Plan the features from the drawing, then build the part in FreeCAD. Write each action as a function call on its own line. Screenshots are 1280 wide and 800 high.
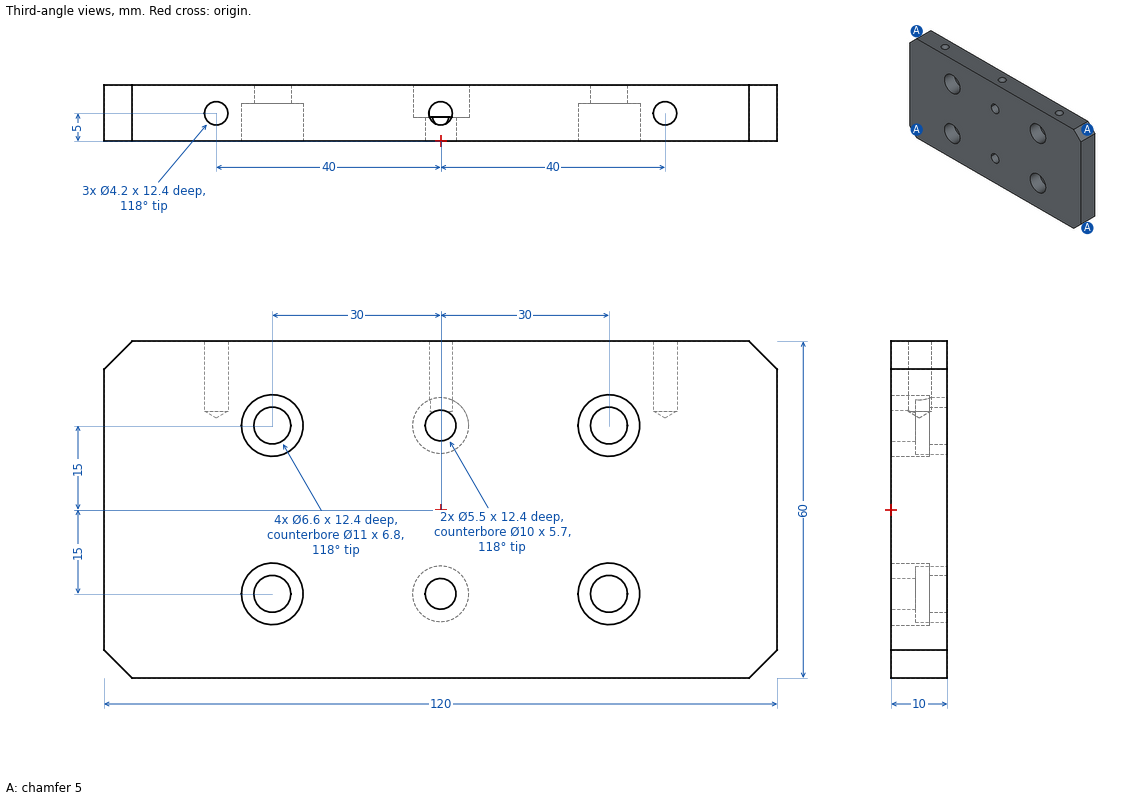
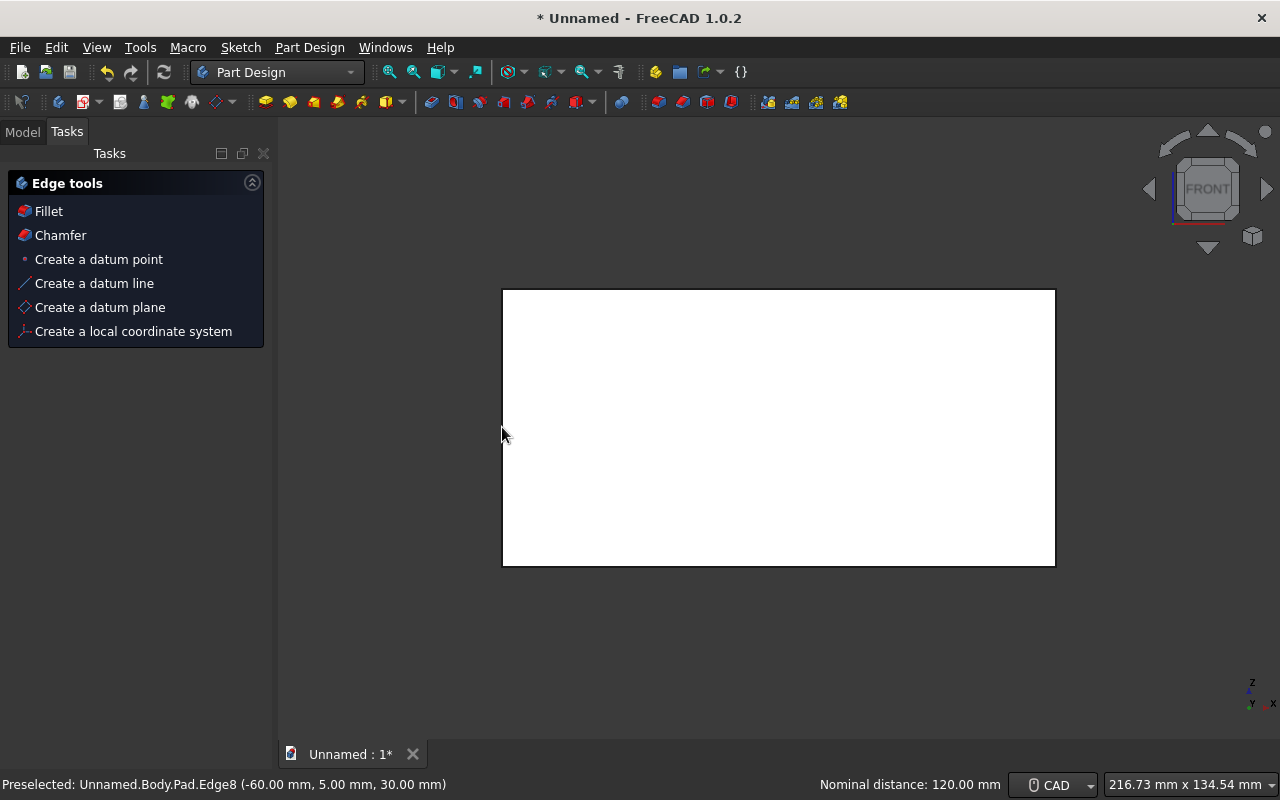
key(3)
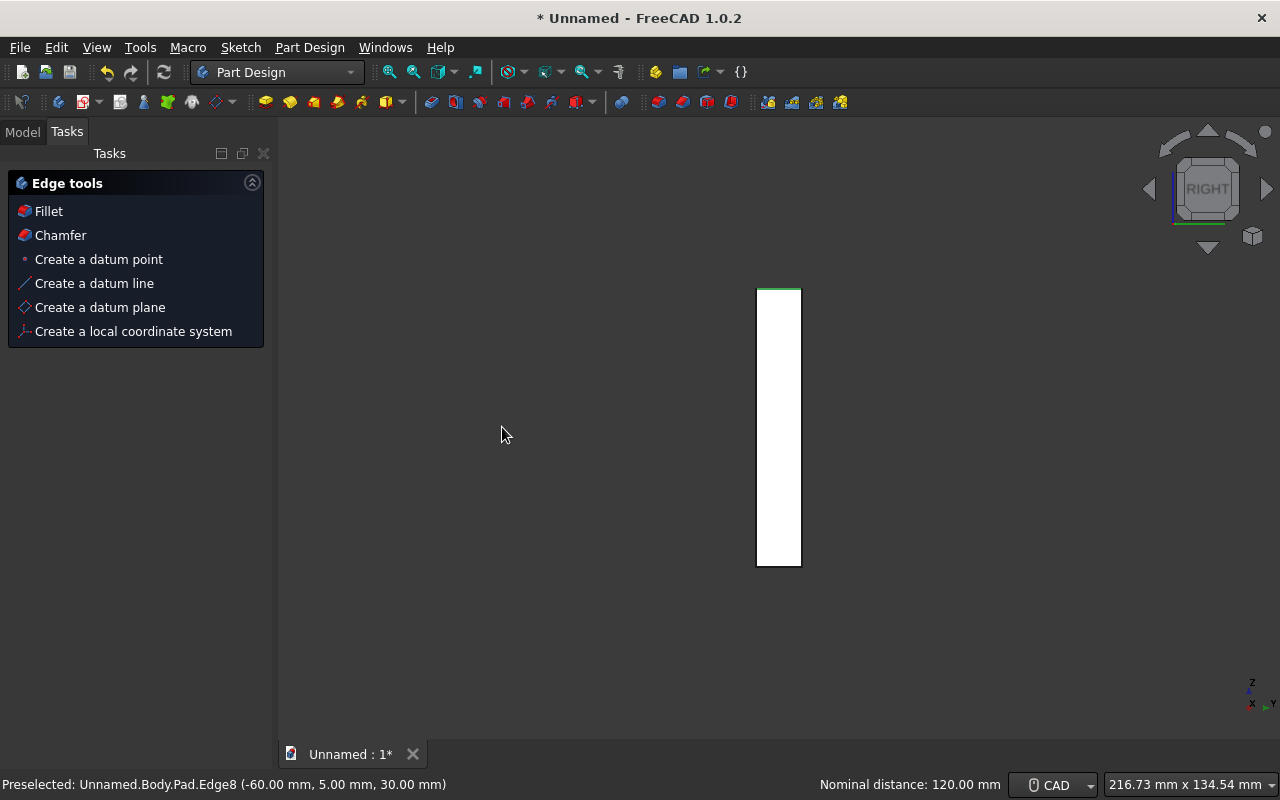
key(v)
key(f)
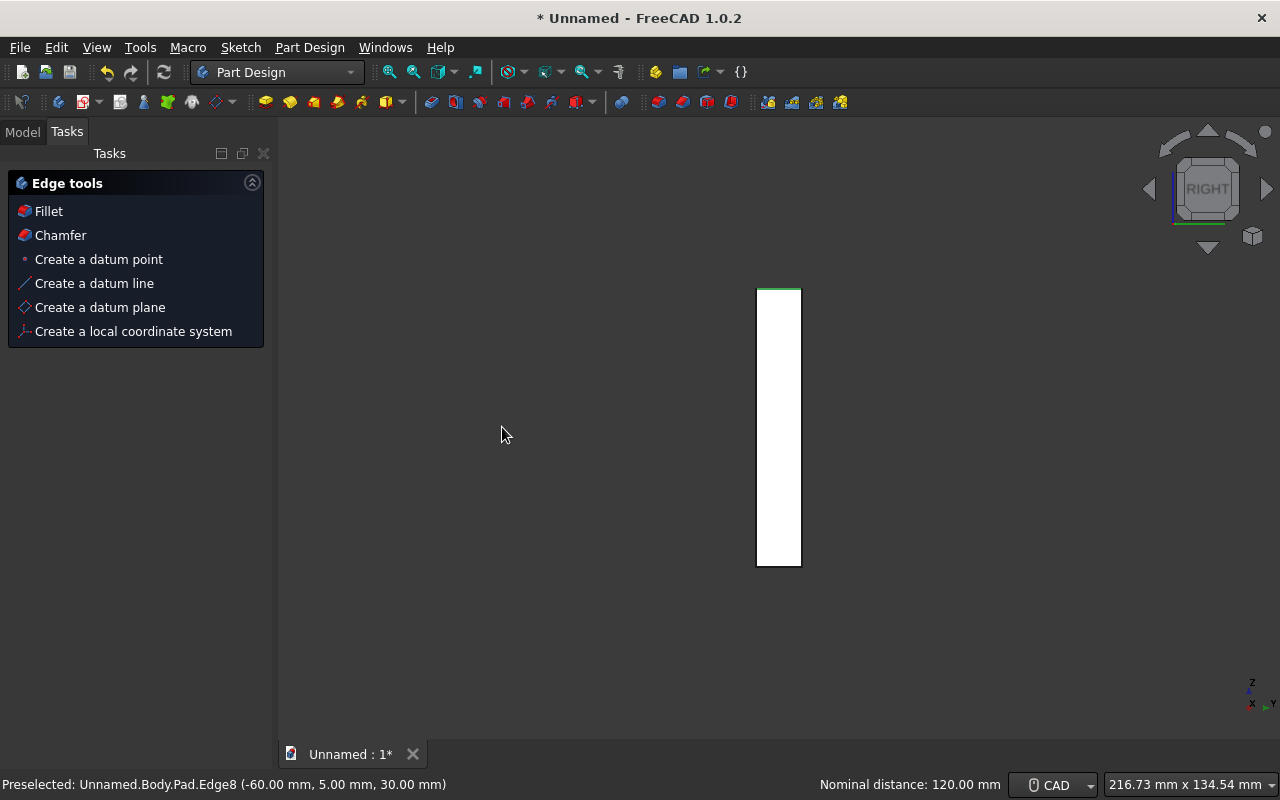
click(779, 566, ctrl)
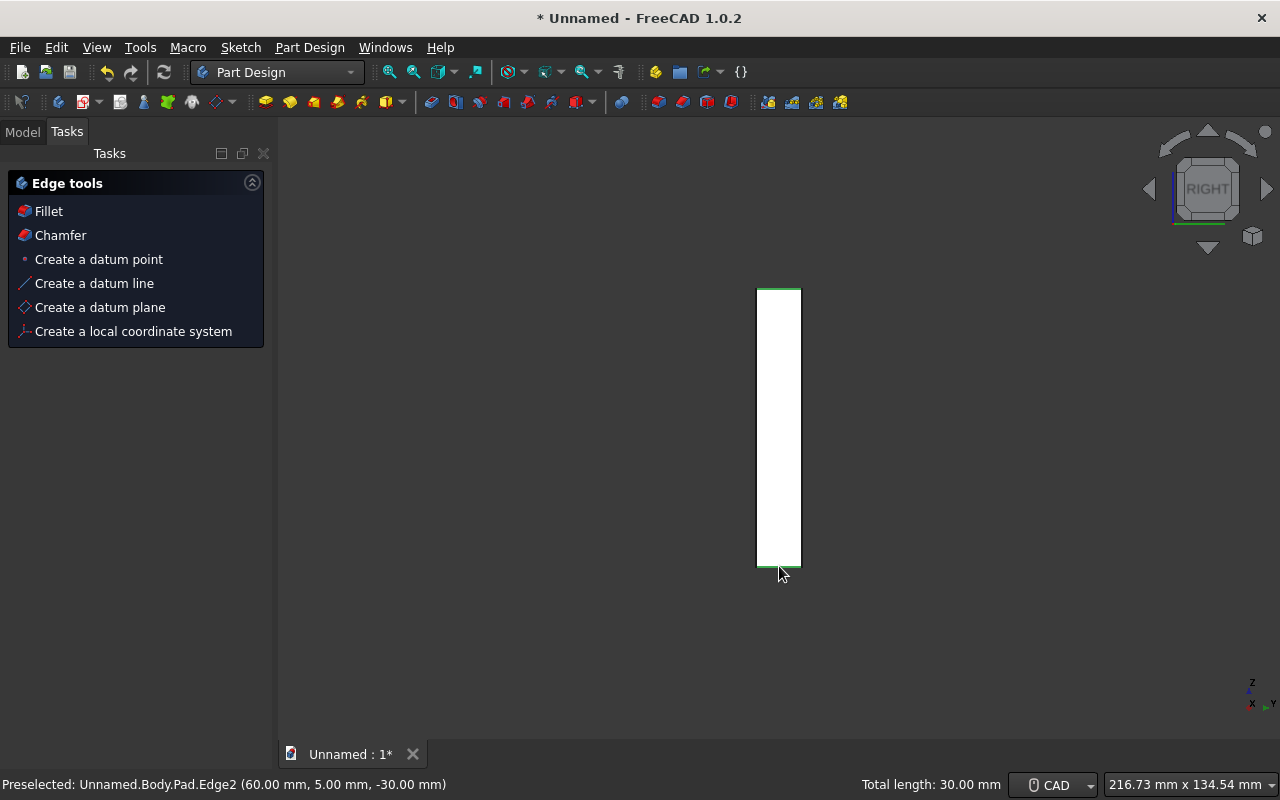
key(5)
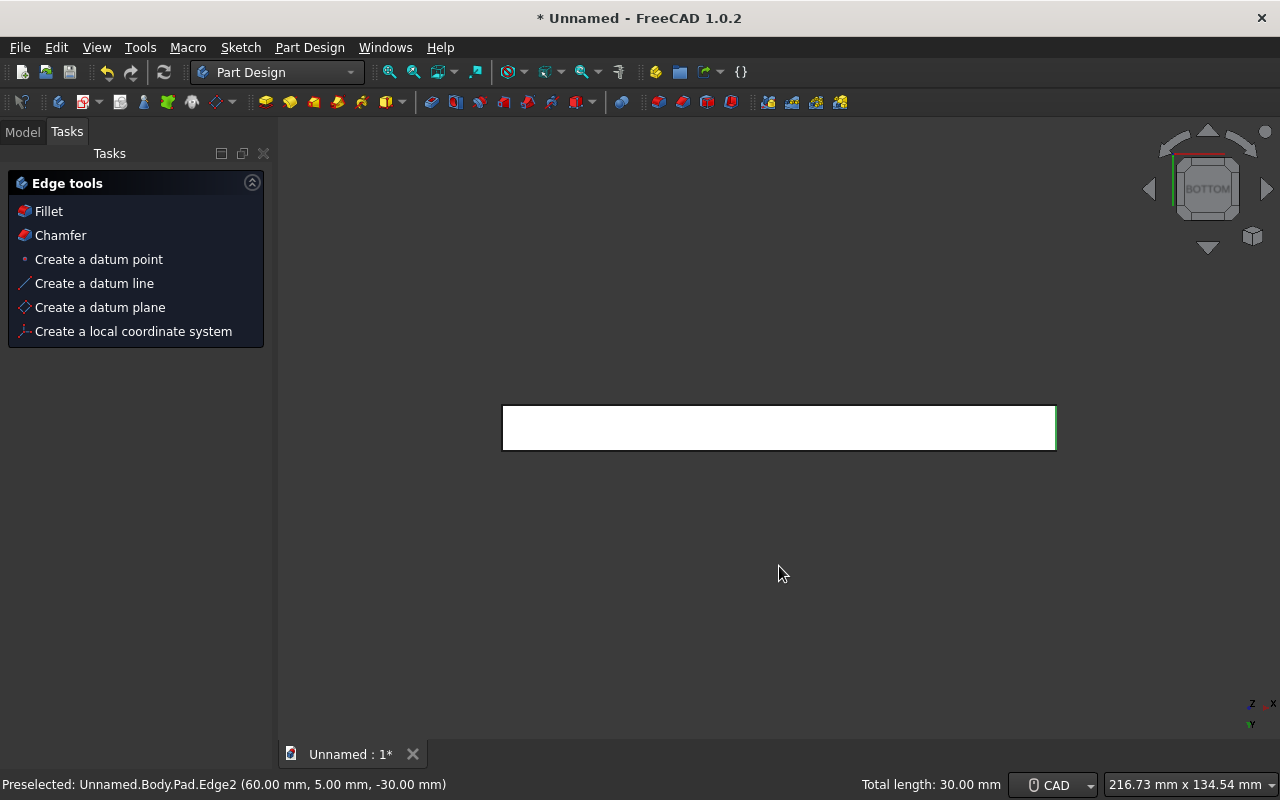
click(502, 427, ctrl)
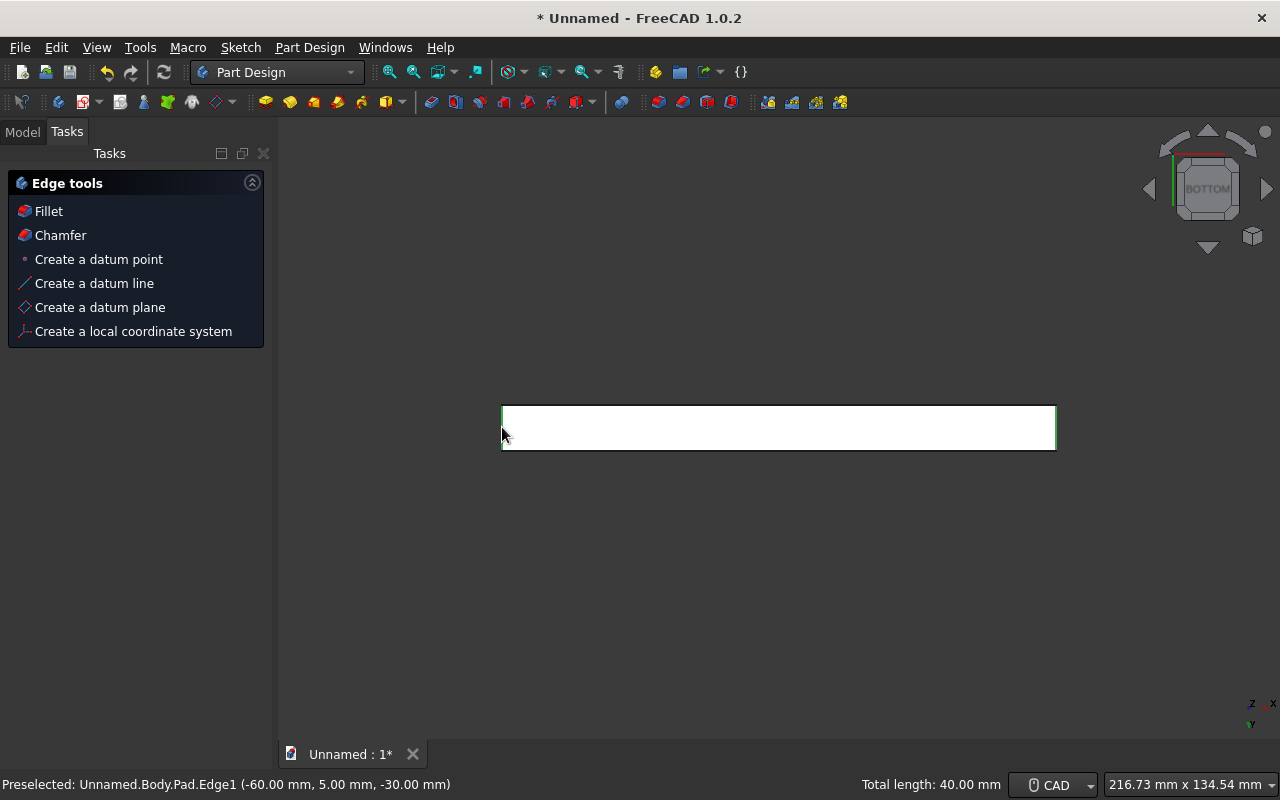
click(684, 102)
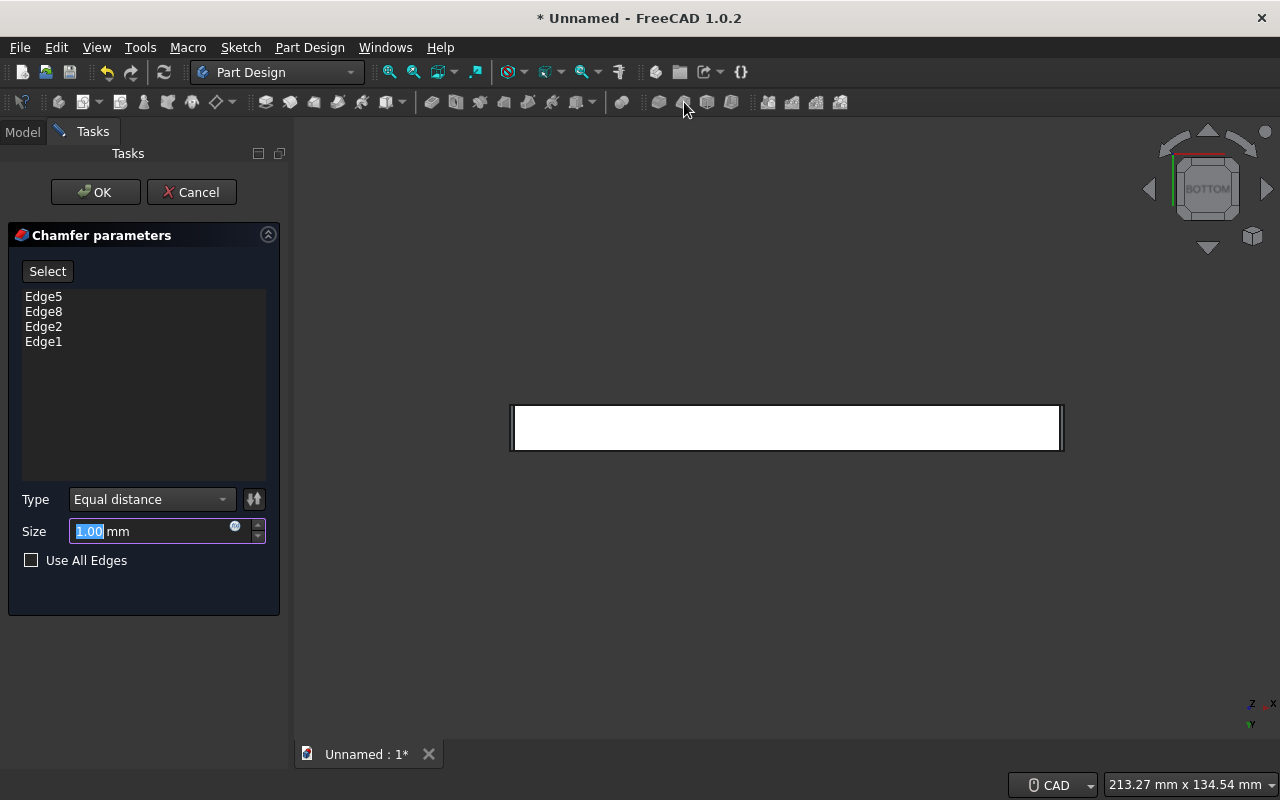
text(5)
key(Tab)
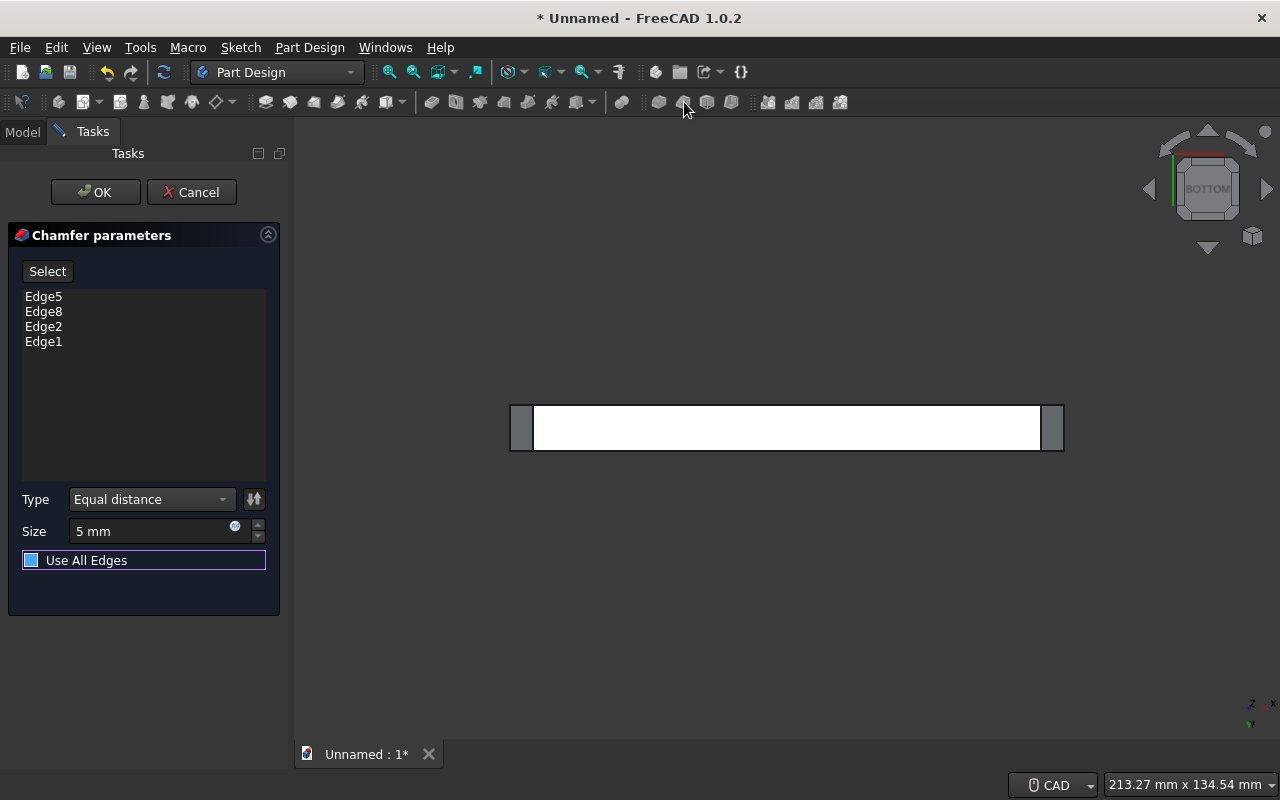
click(96, 192)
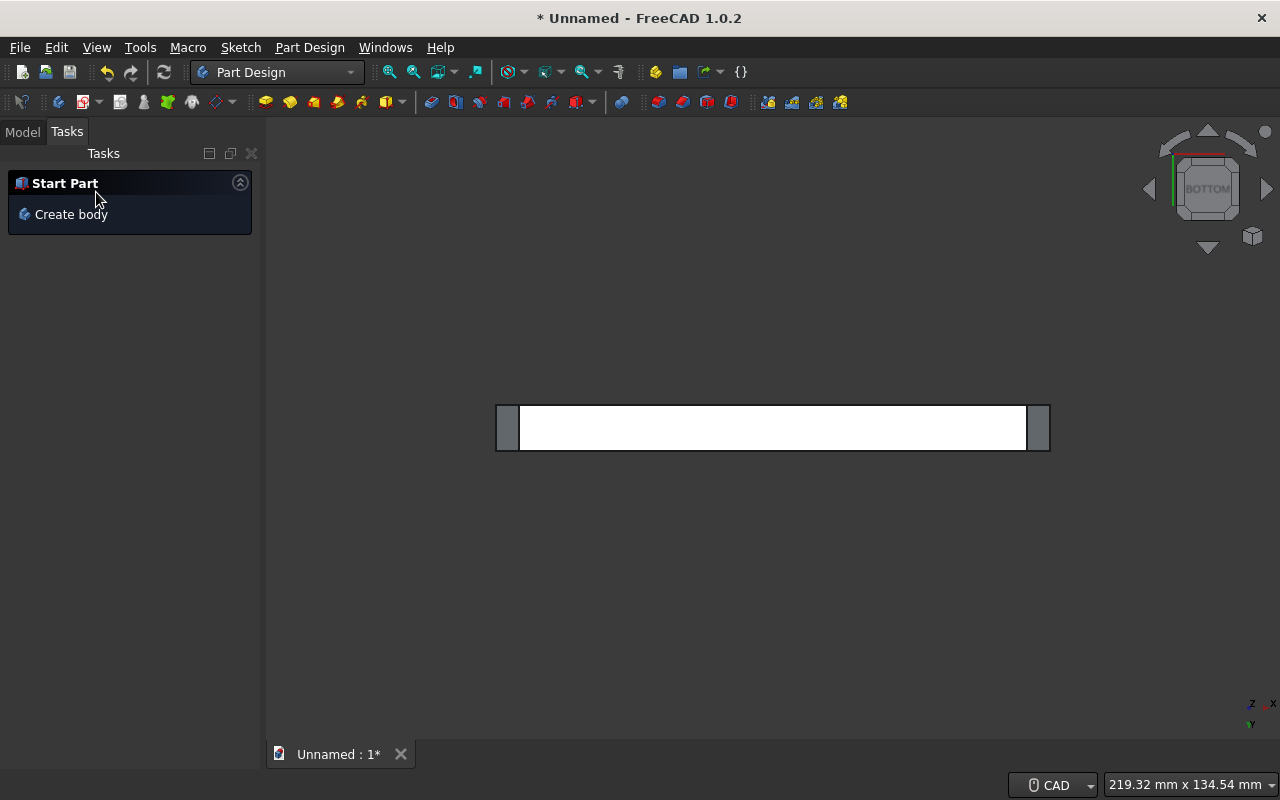
key(0)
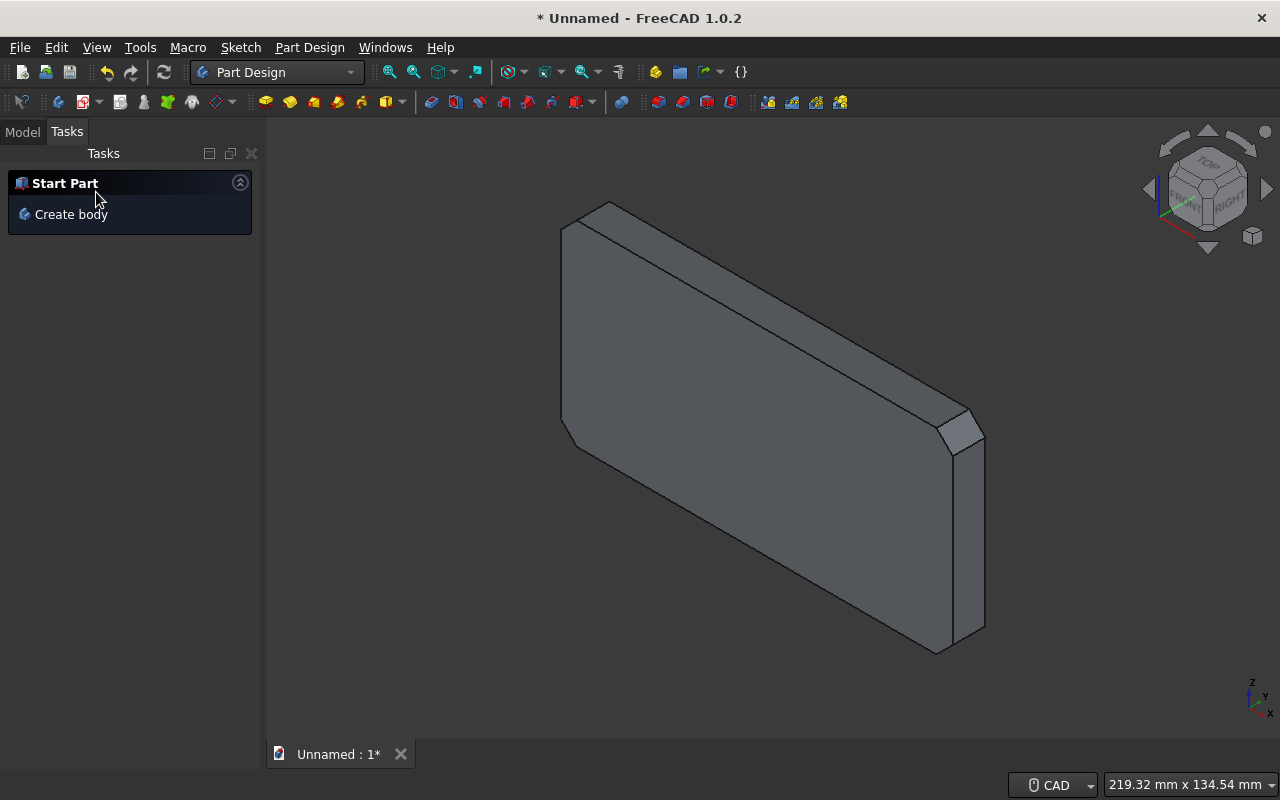
click(927, 403)